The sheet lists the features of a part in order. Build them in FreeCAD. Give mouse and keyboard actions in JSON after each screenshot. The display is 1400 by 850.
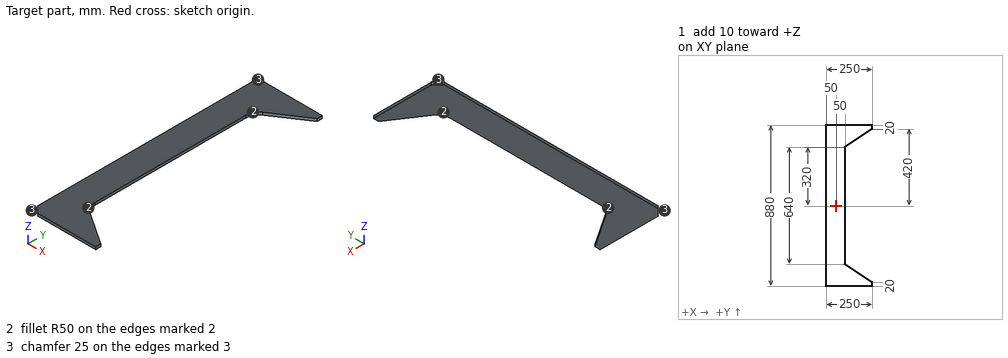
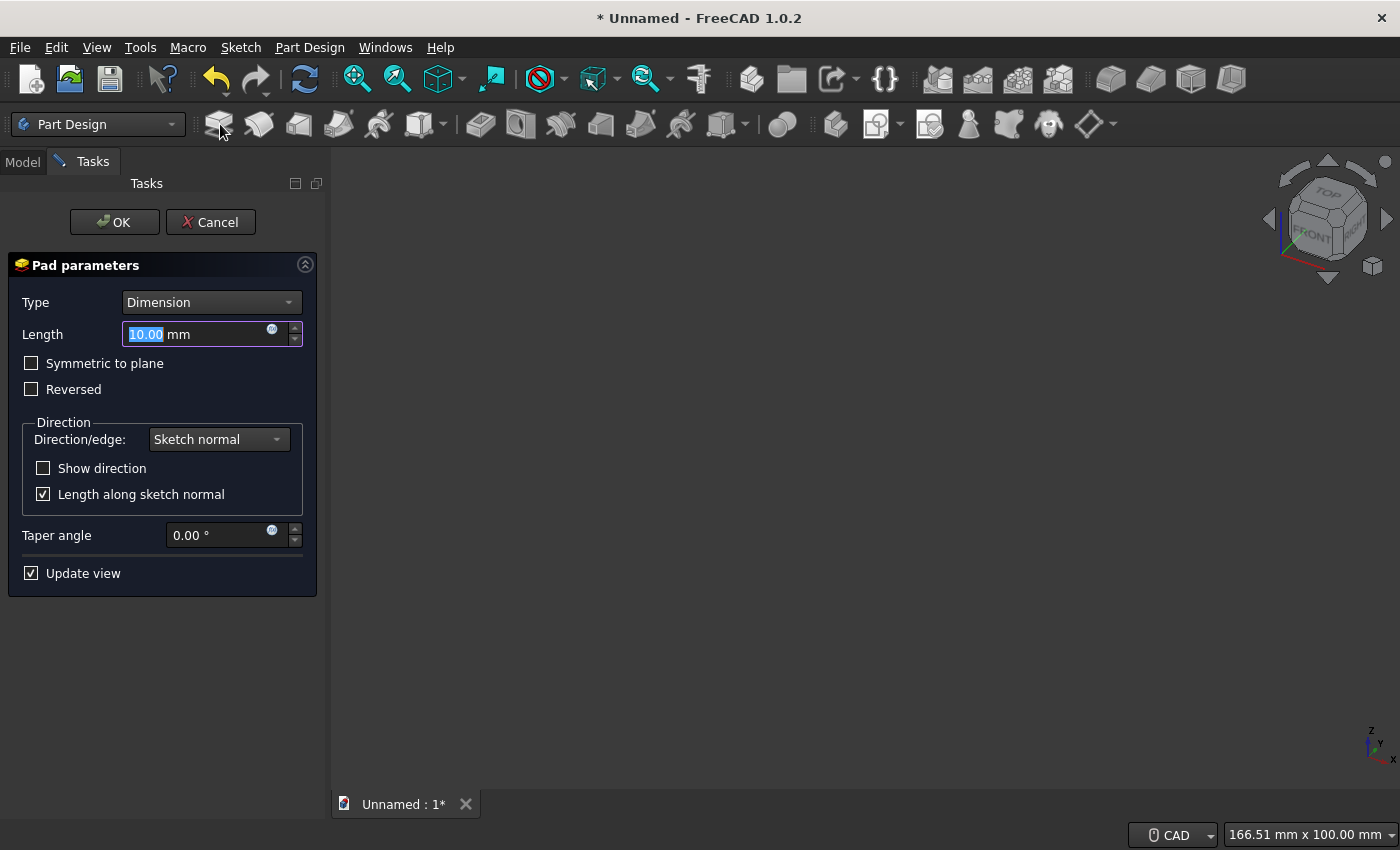
{"action": "type", "text": "10"}
{"action": "key", "text": "Tab"}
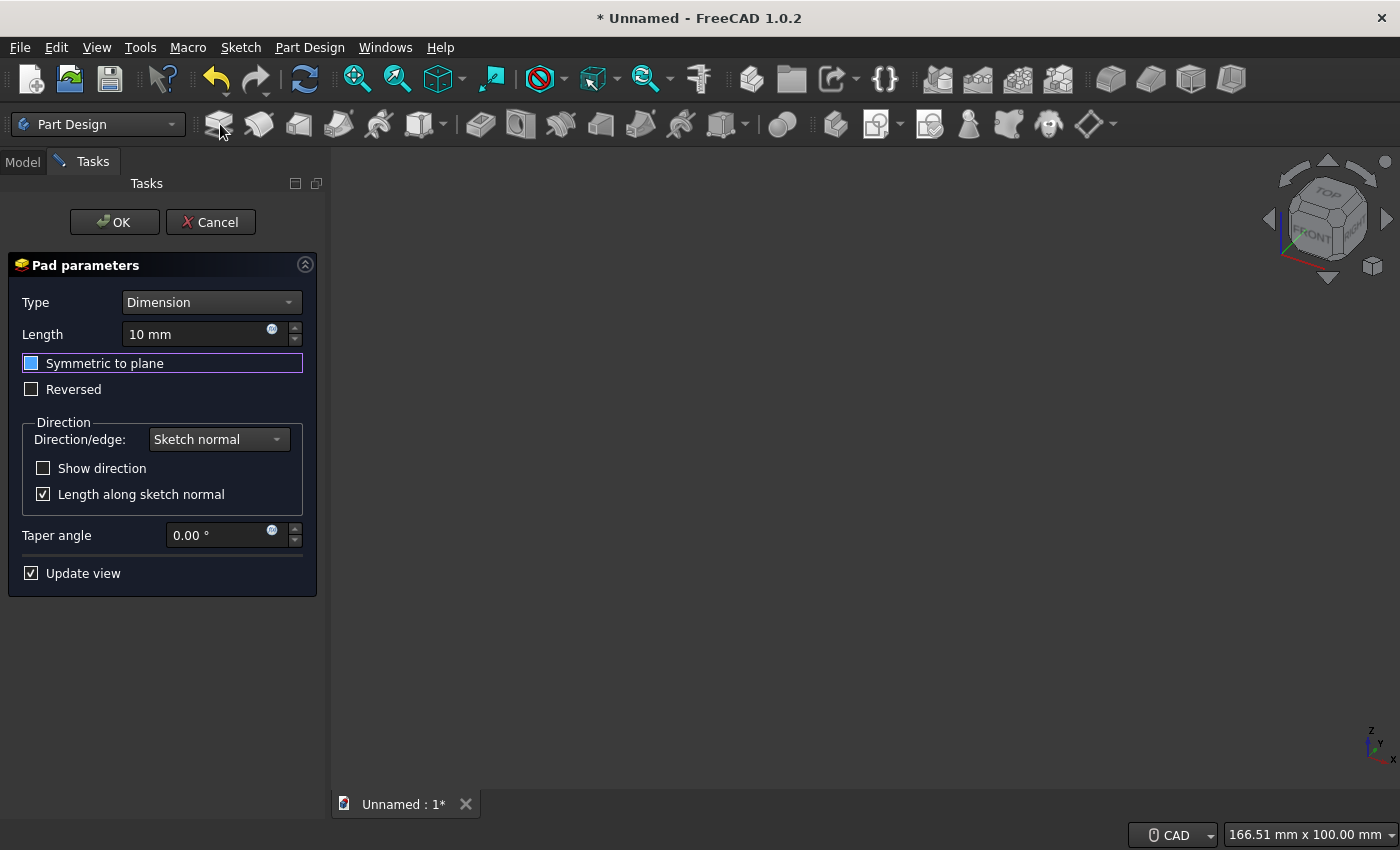
{"action": "left_click", "coordinate": [115, 222]}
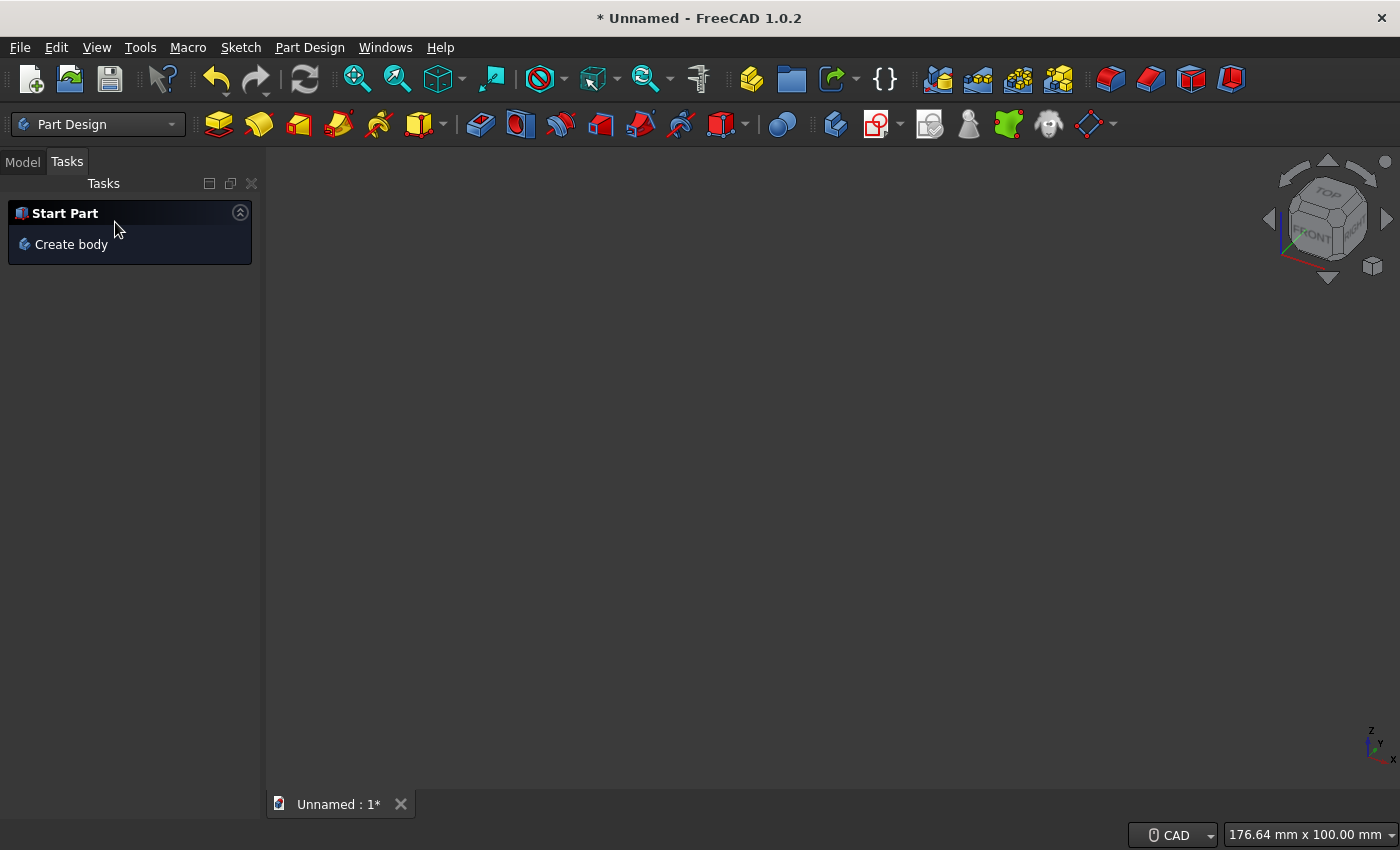
{"action": "key", "text": "v f"}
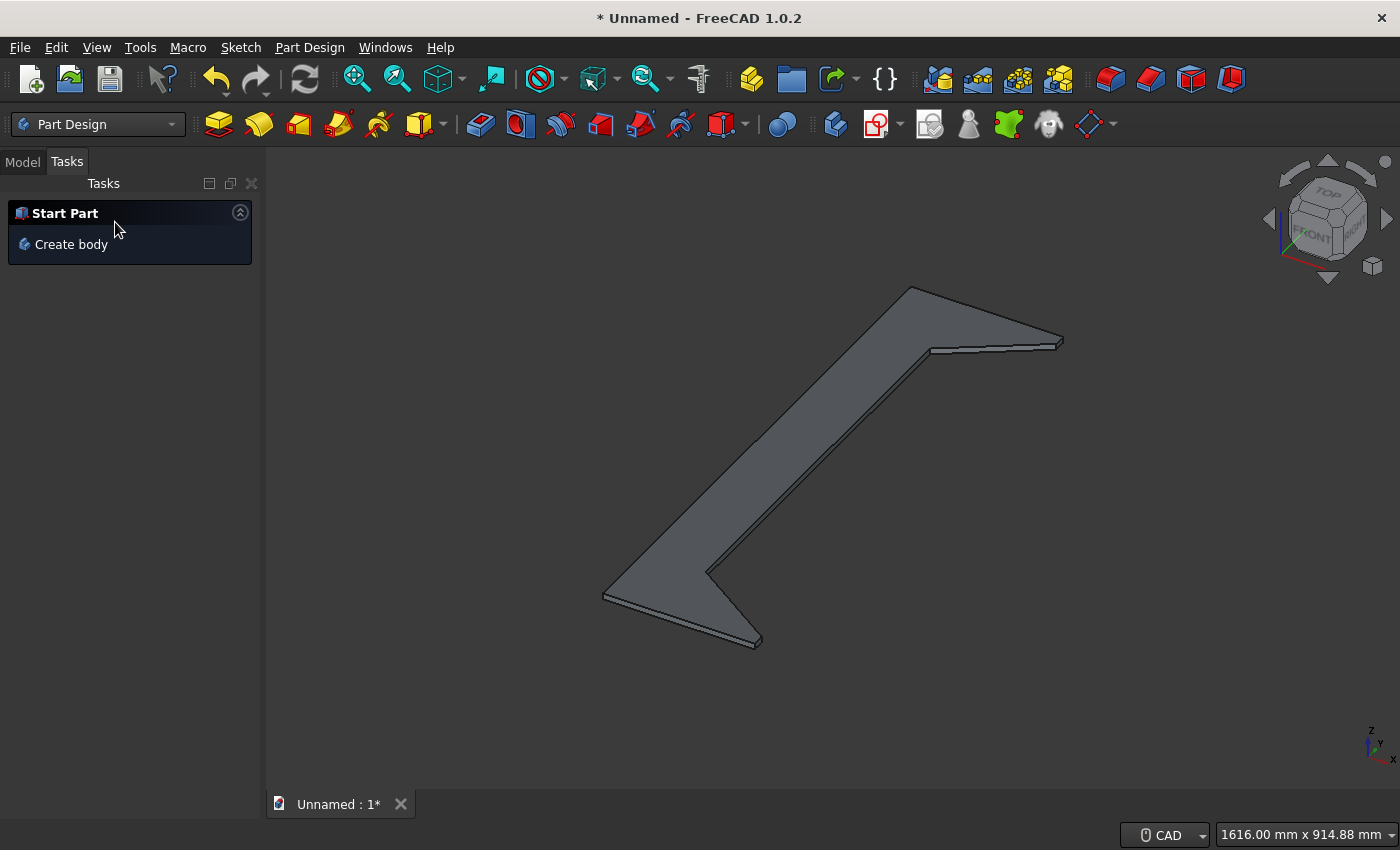
{"action": "scroll", "coordinate": [930, 350], "scroll_direction": "up", "scroll_amount": 9}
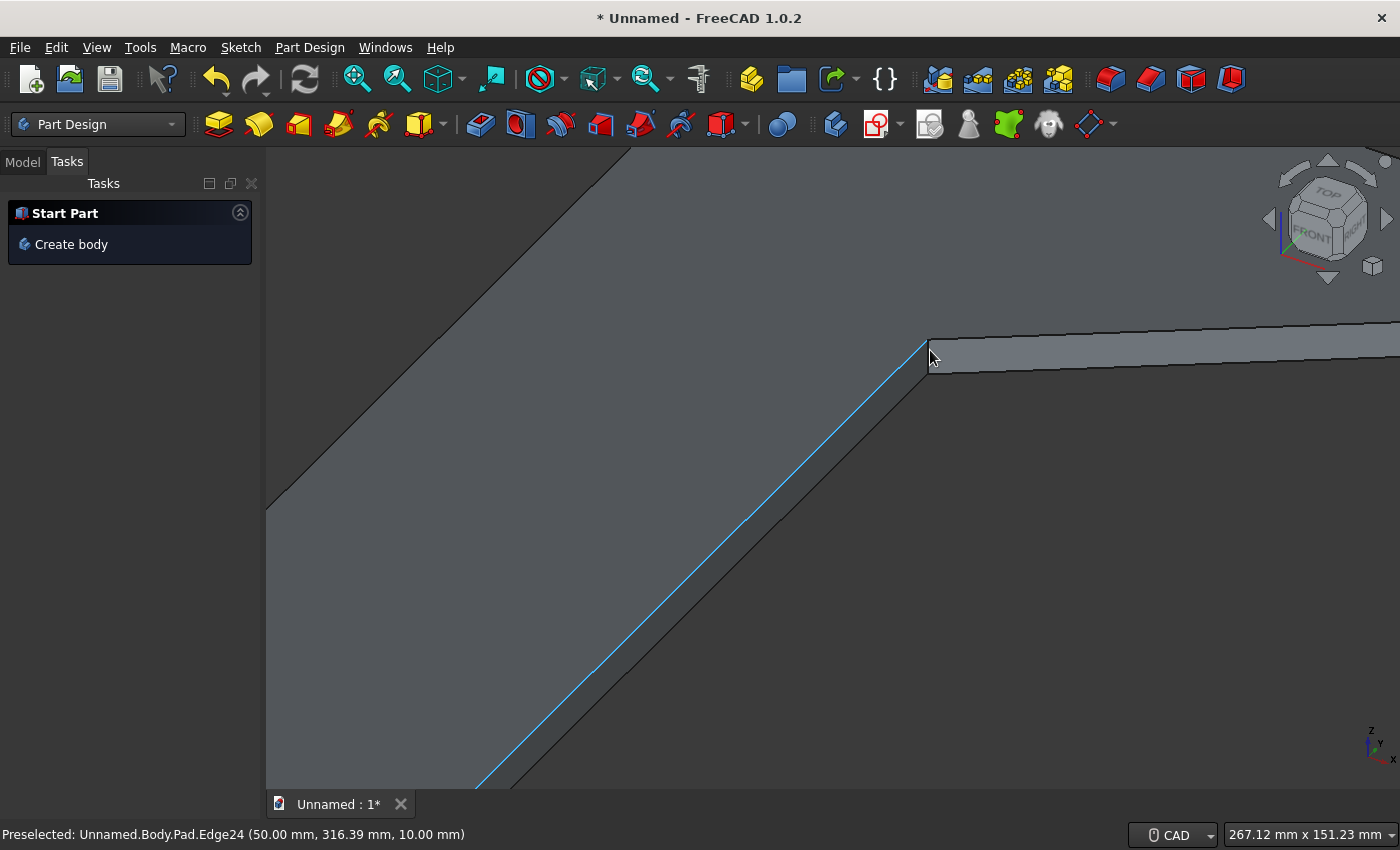
{"action": "key", "text": "v f"}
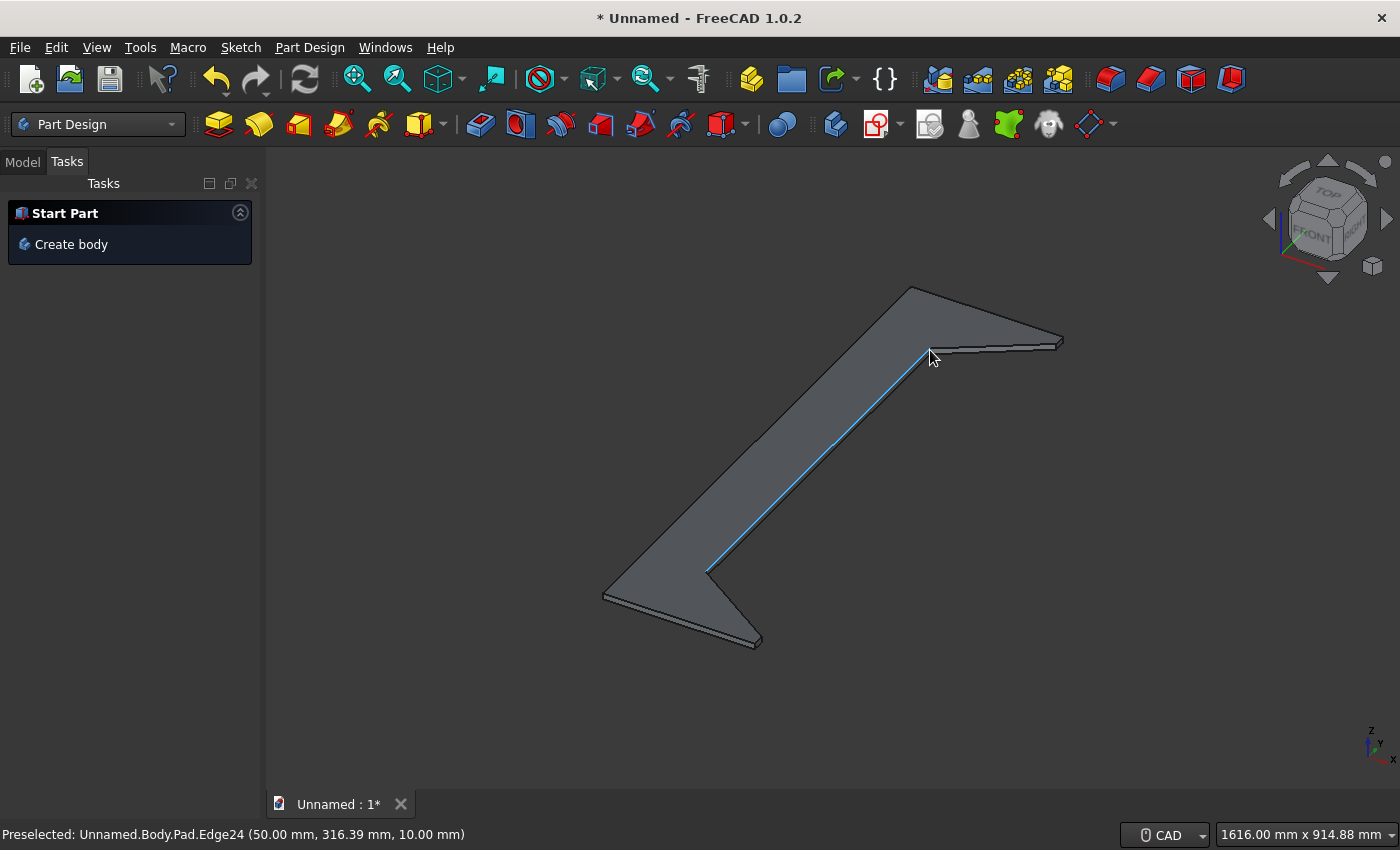
{"action": "key", "text": "0"}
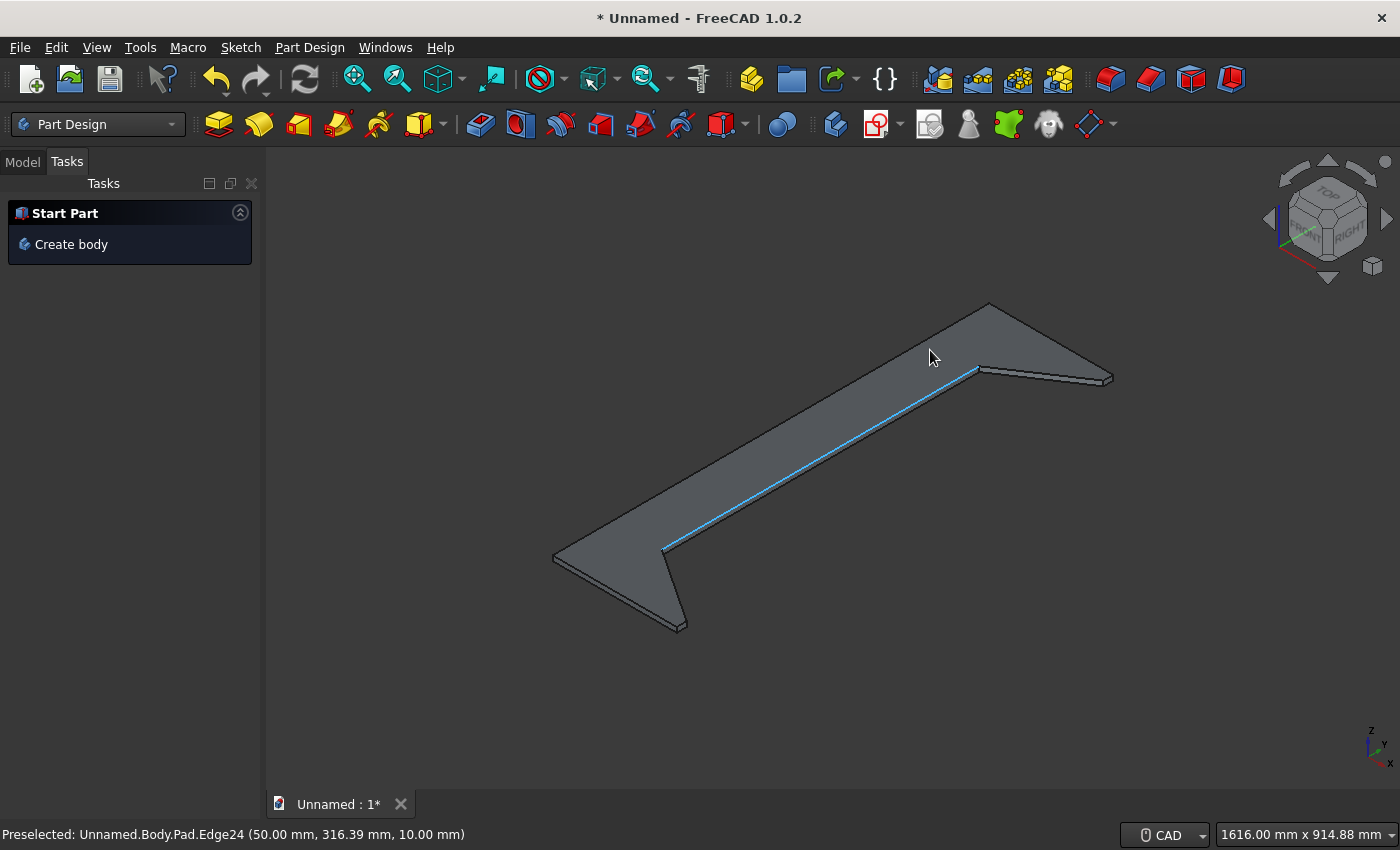
{"action": "scroll", "coordinate": [979, 368], "scroll_direction": "up", "scroll_amount": 9}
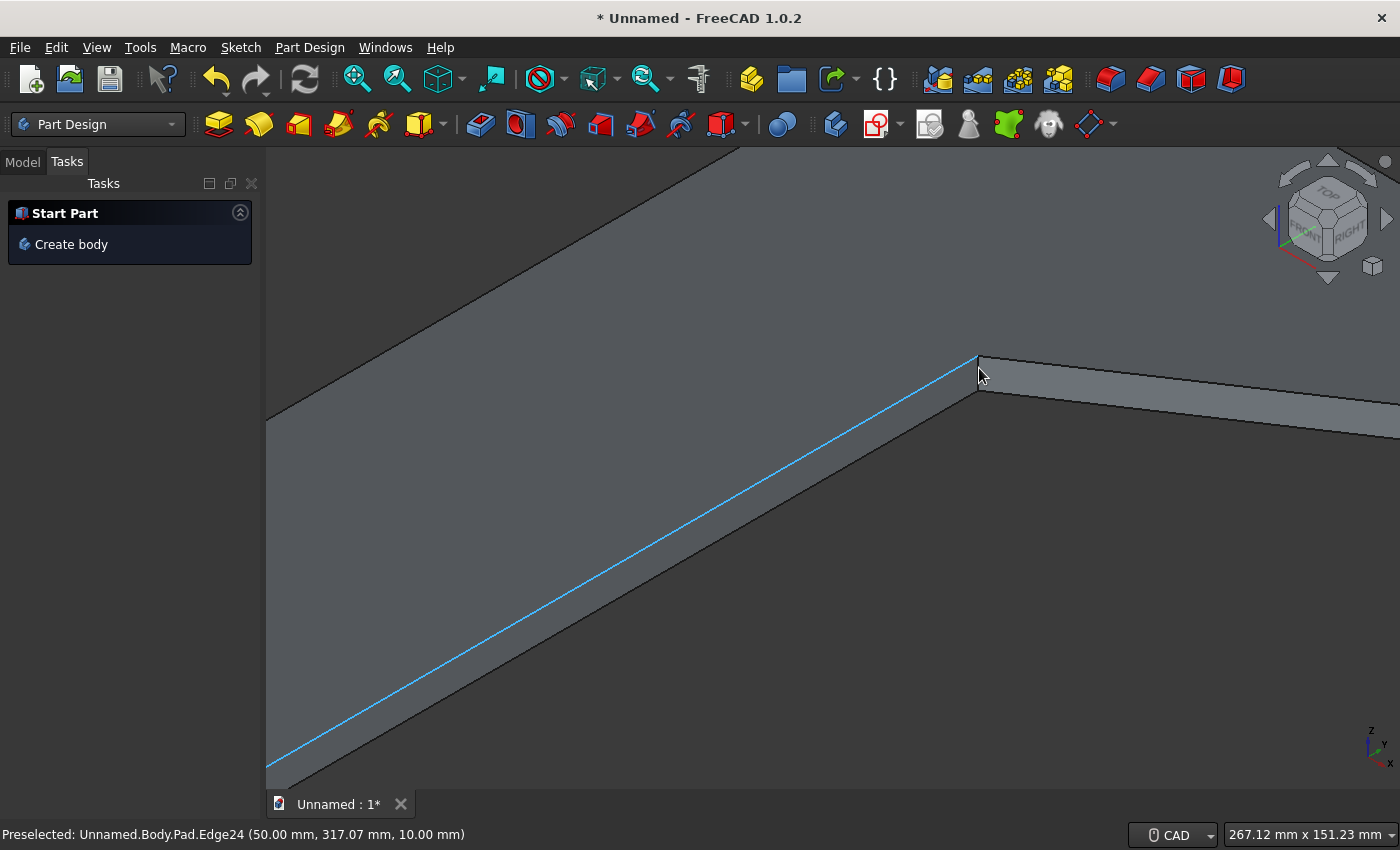
{"action": "key", "text": "v f"}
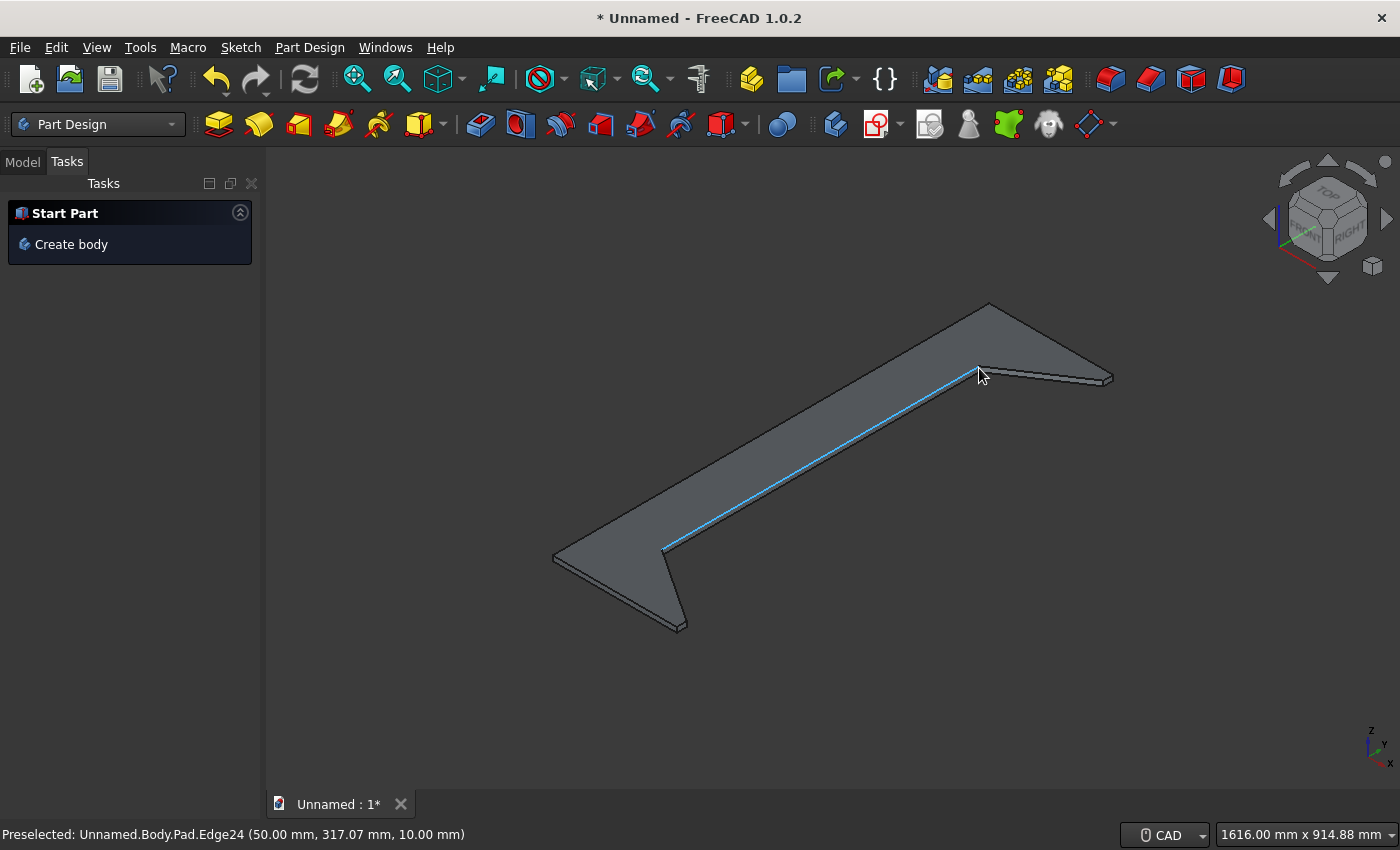
{"action": "key", "text": "2"}